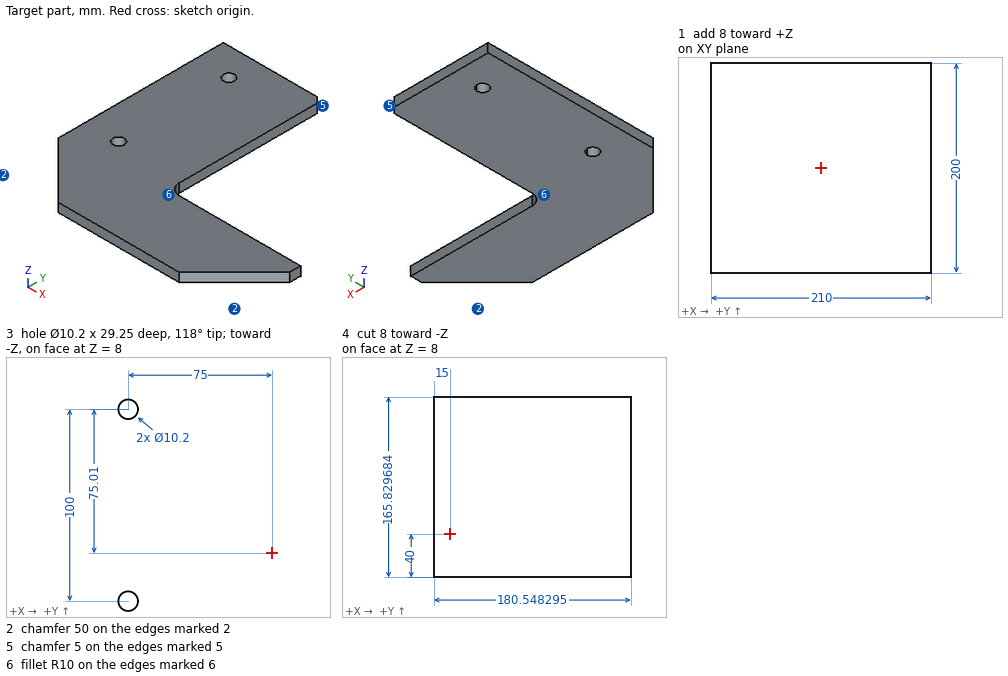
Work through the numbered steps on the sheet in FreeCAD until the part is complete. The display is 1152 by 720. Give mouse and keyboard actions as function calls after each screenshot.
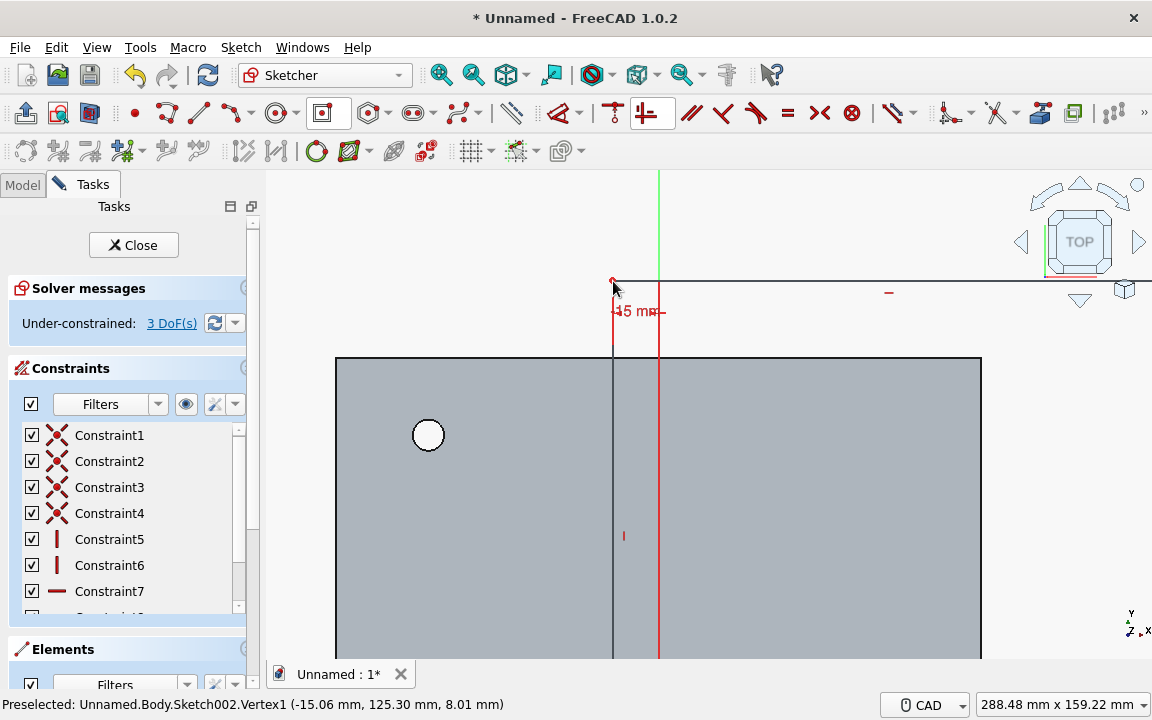
scroll(337, 269, down, 3)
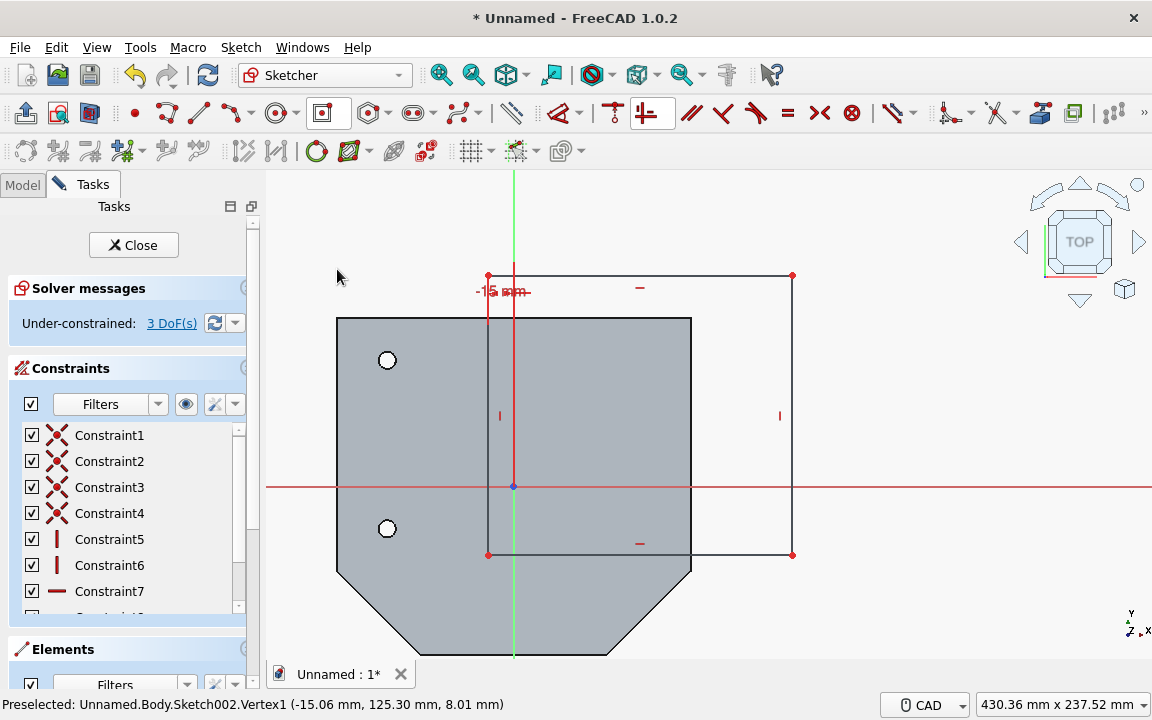
click(488, 555)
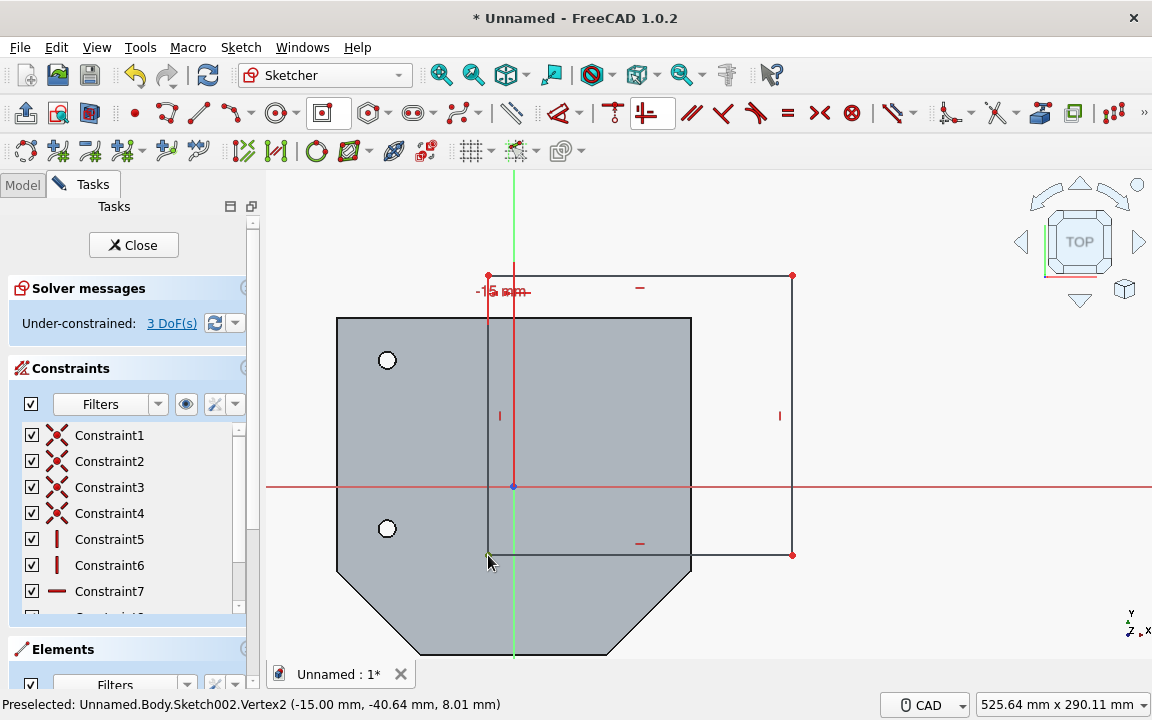
key(i)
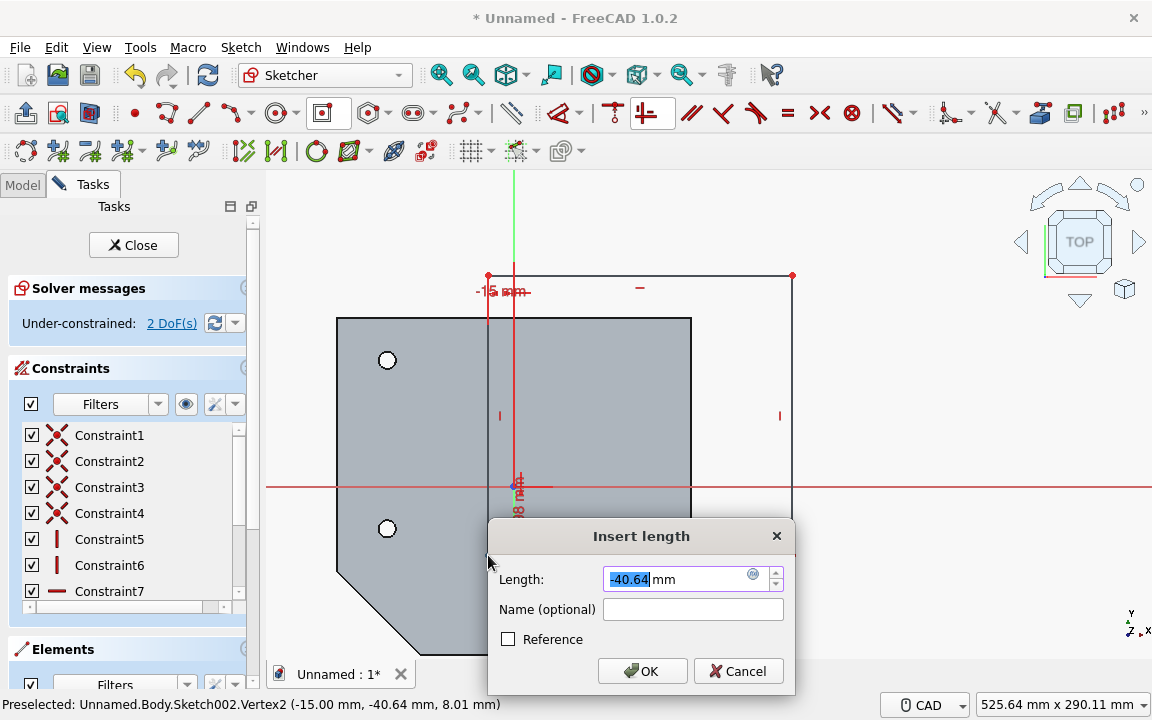
text(-40)
key(Return)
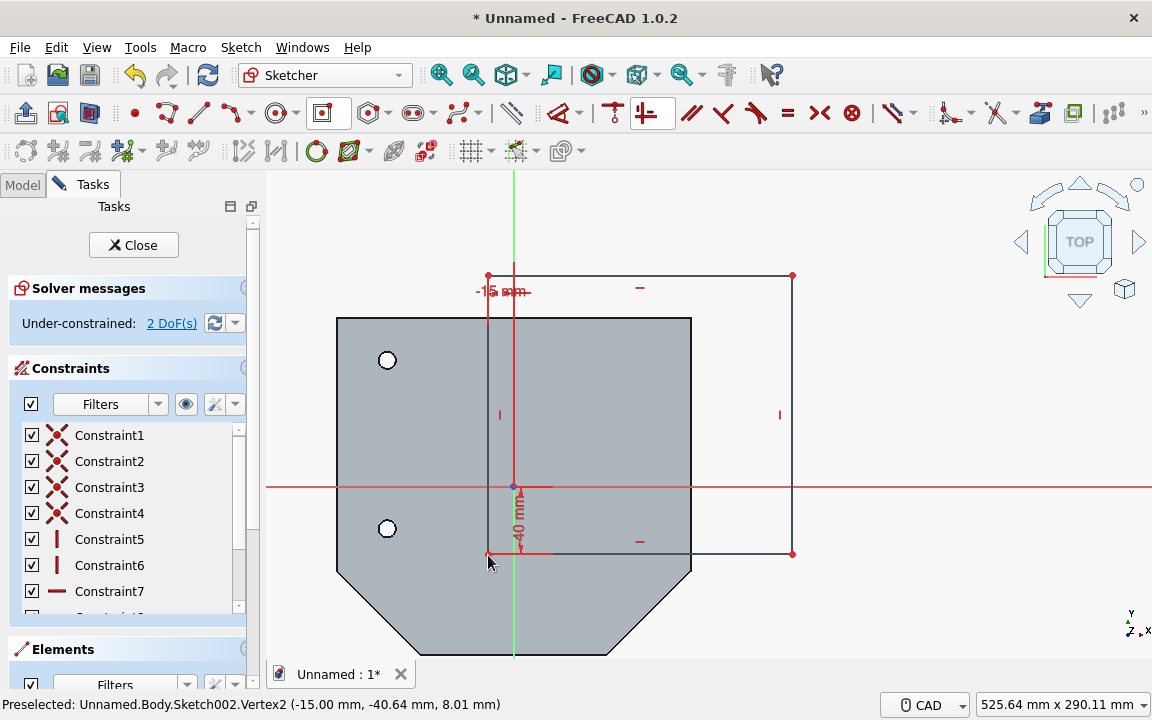
click(488, 359)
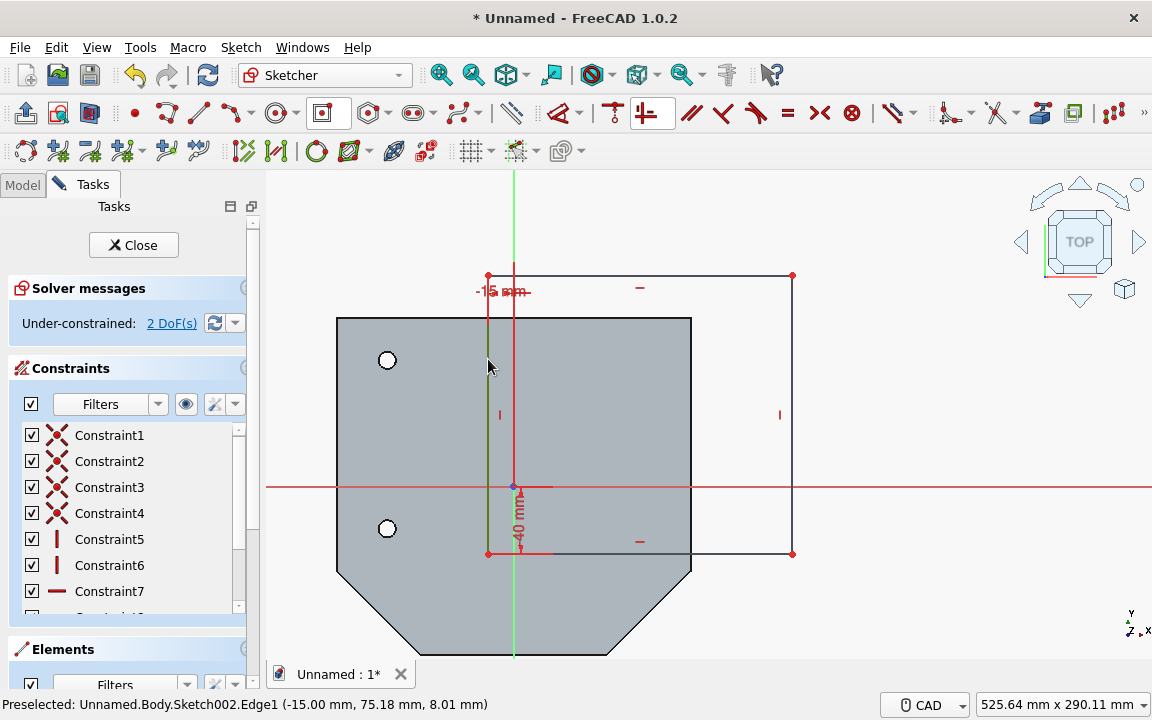
key(i)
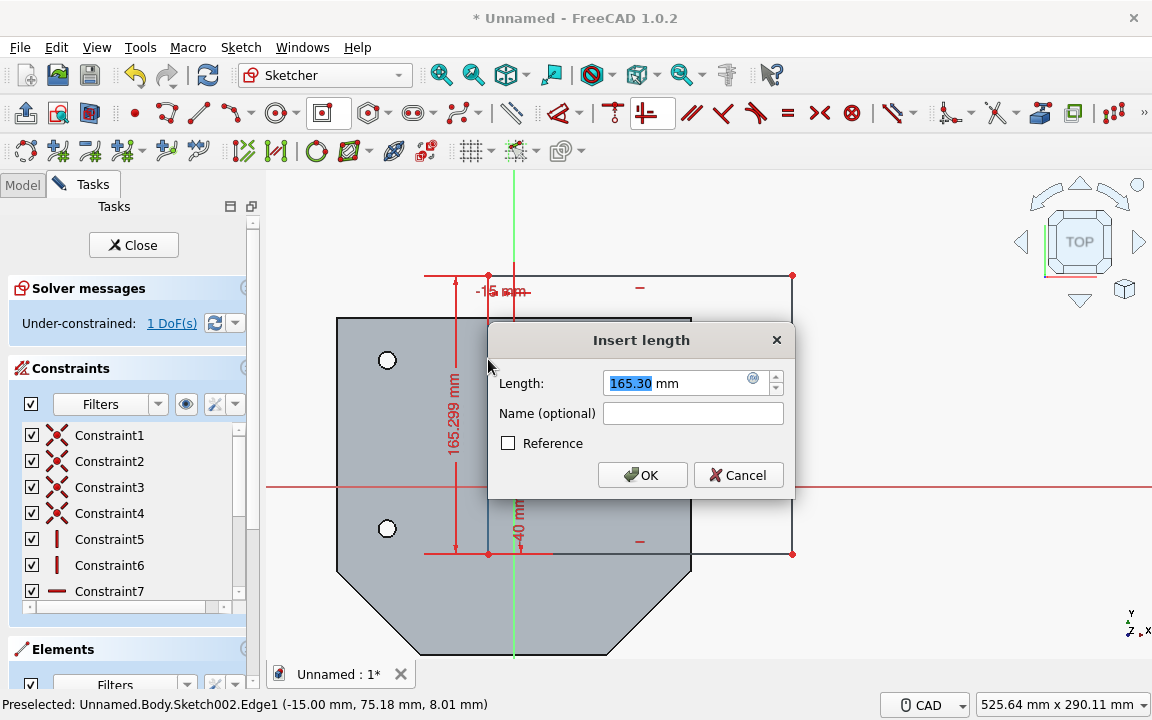
text(165.829684)
key(Return)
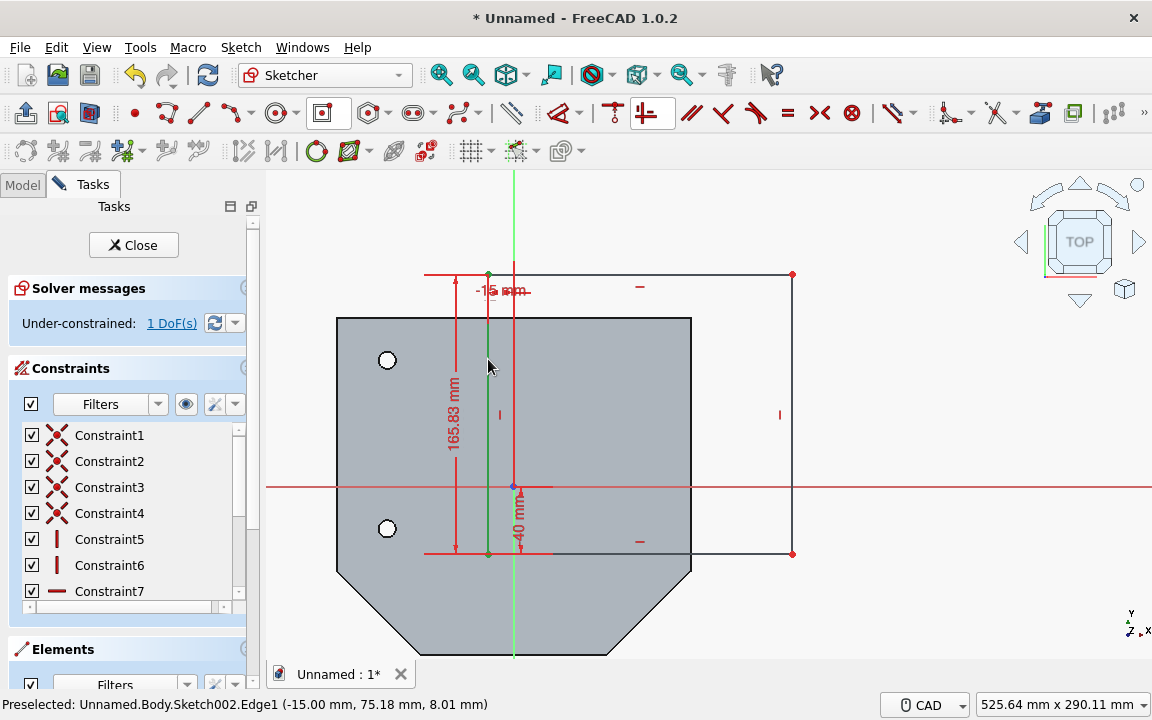
click(580, 554)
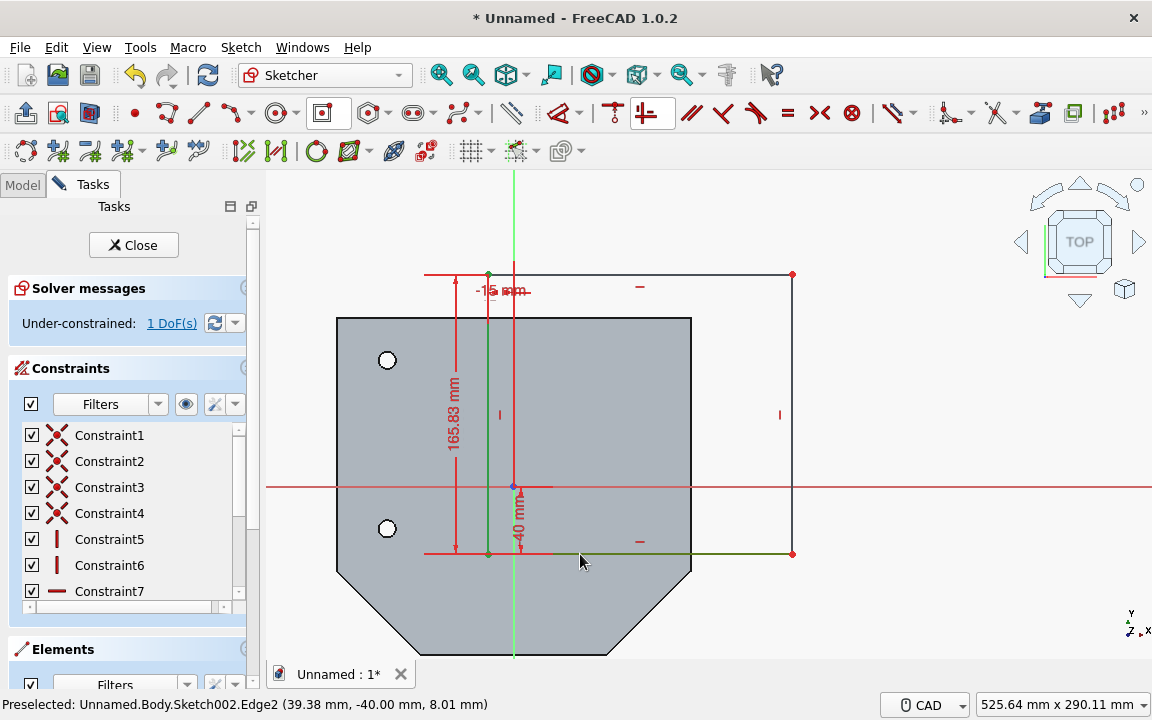
key(l)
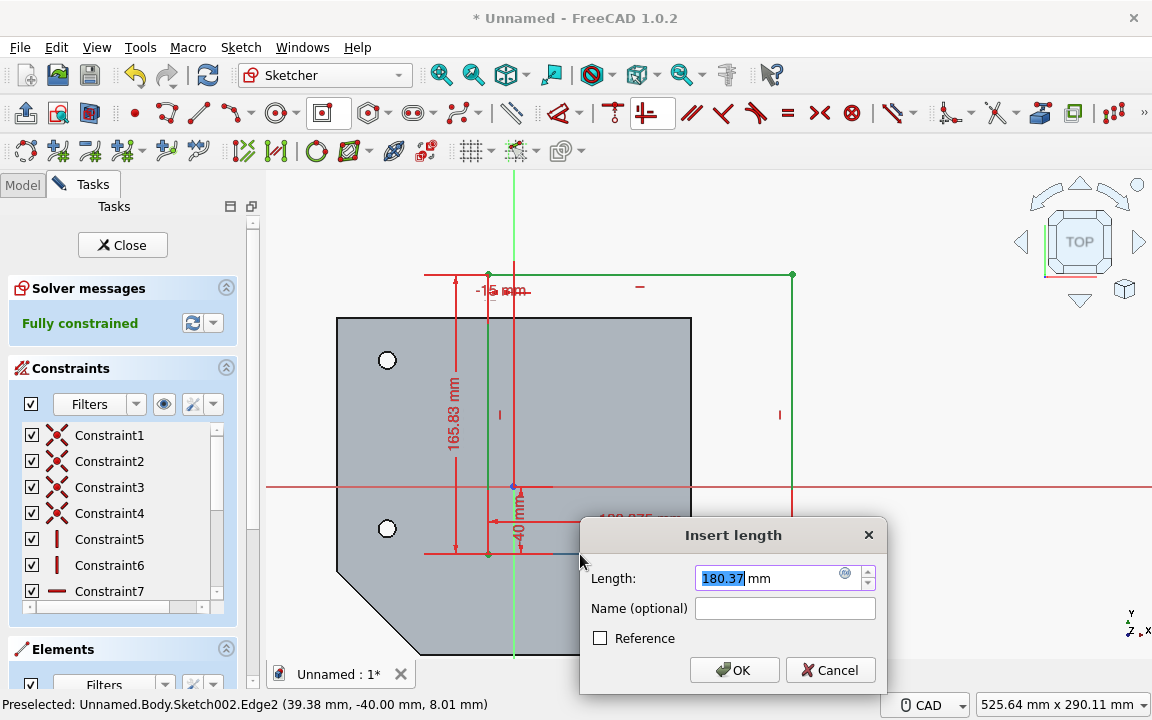
text(180.548295)
key(Return)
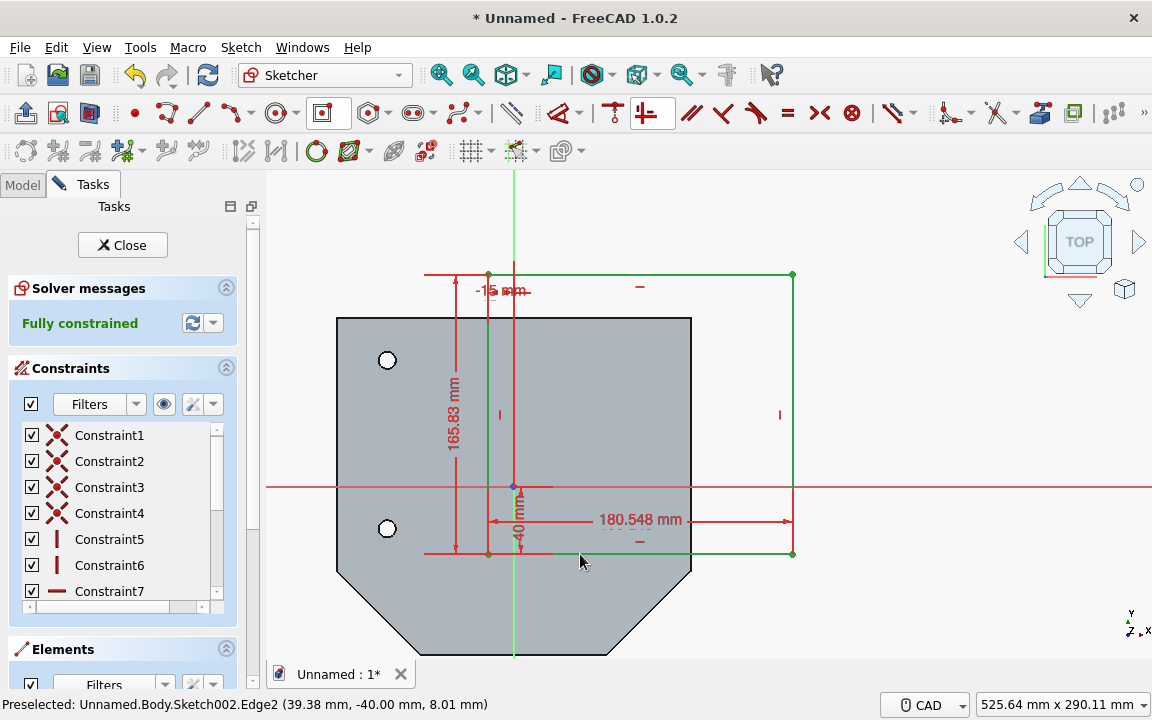
click(123, 245)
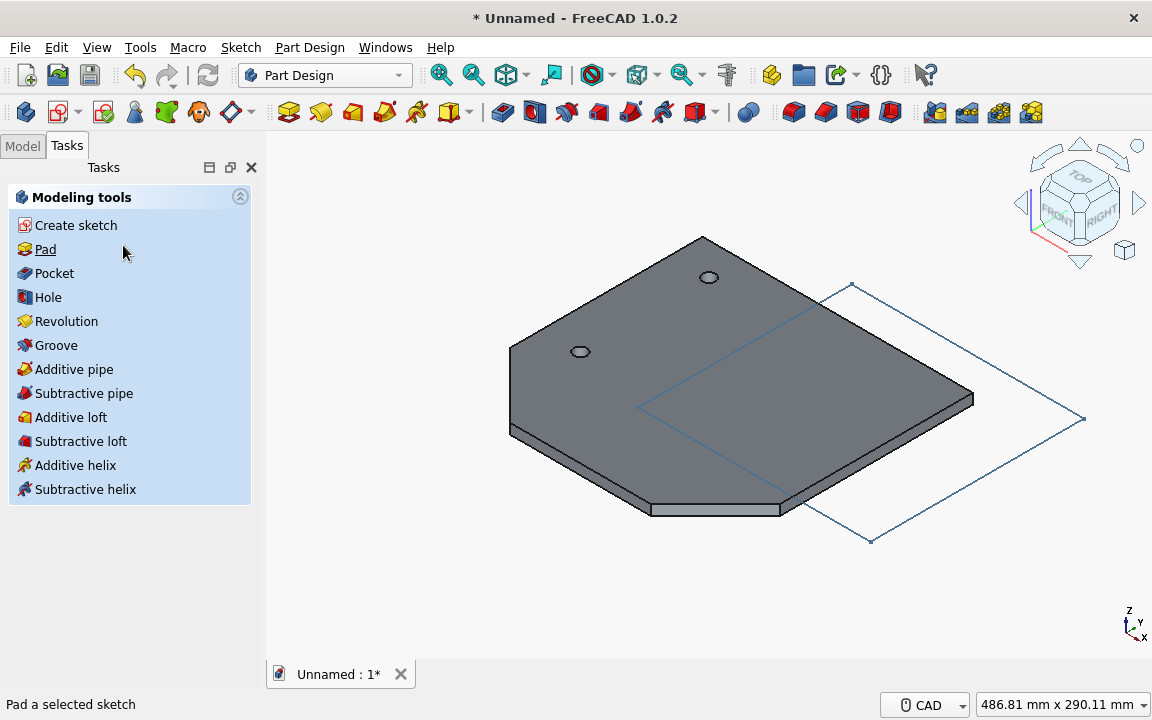
click(504, 112)